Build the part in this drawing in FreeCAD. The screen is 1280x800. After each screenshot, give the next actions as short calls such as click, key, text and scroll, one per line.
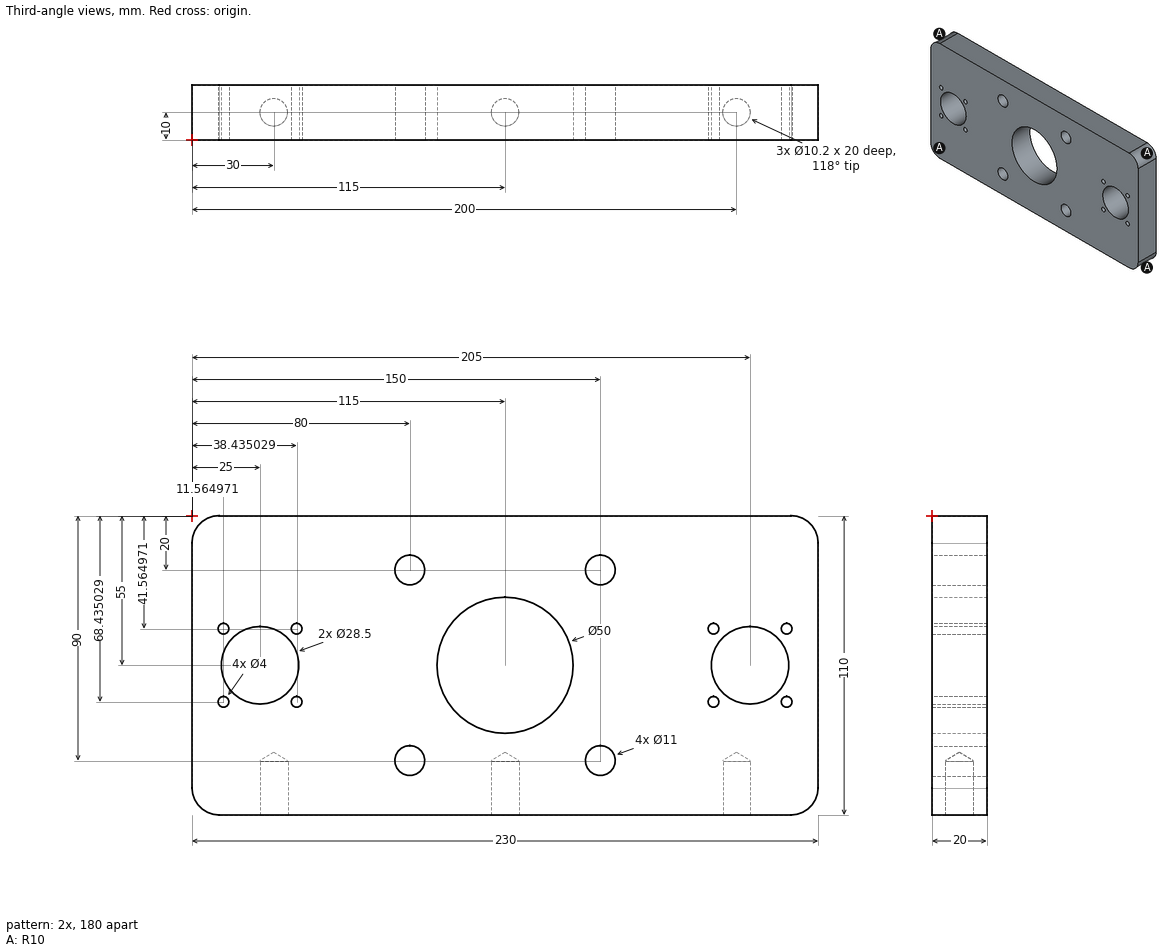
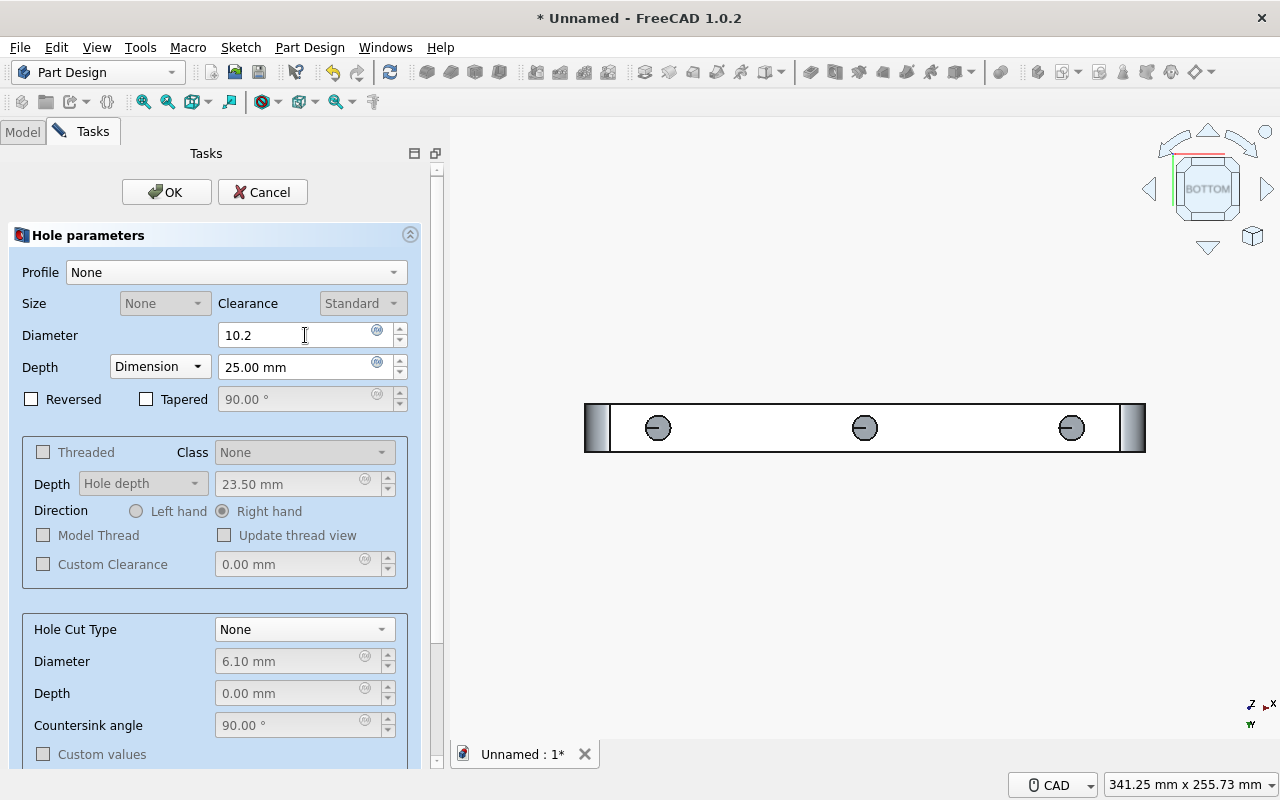
triple_click(305, 367)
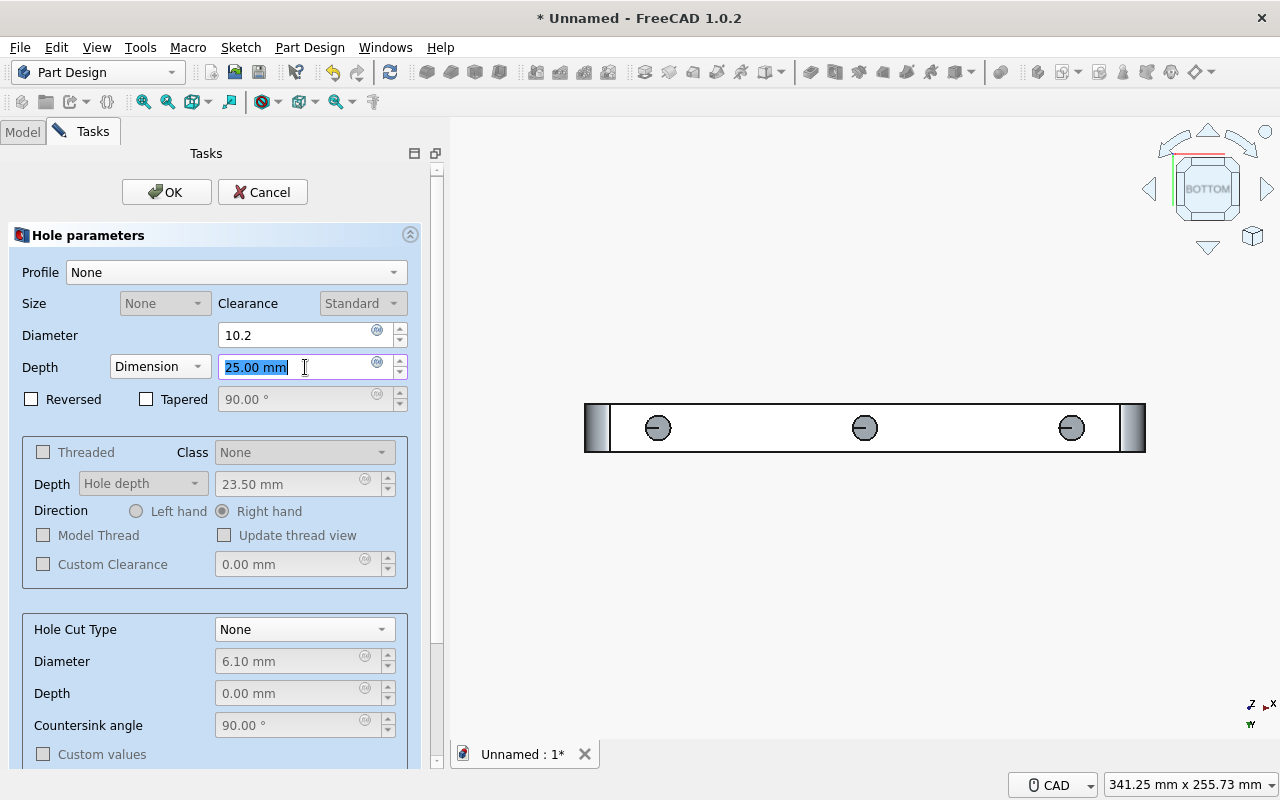
text(20)
key(Tab)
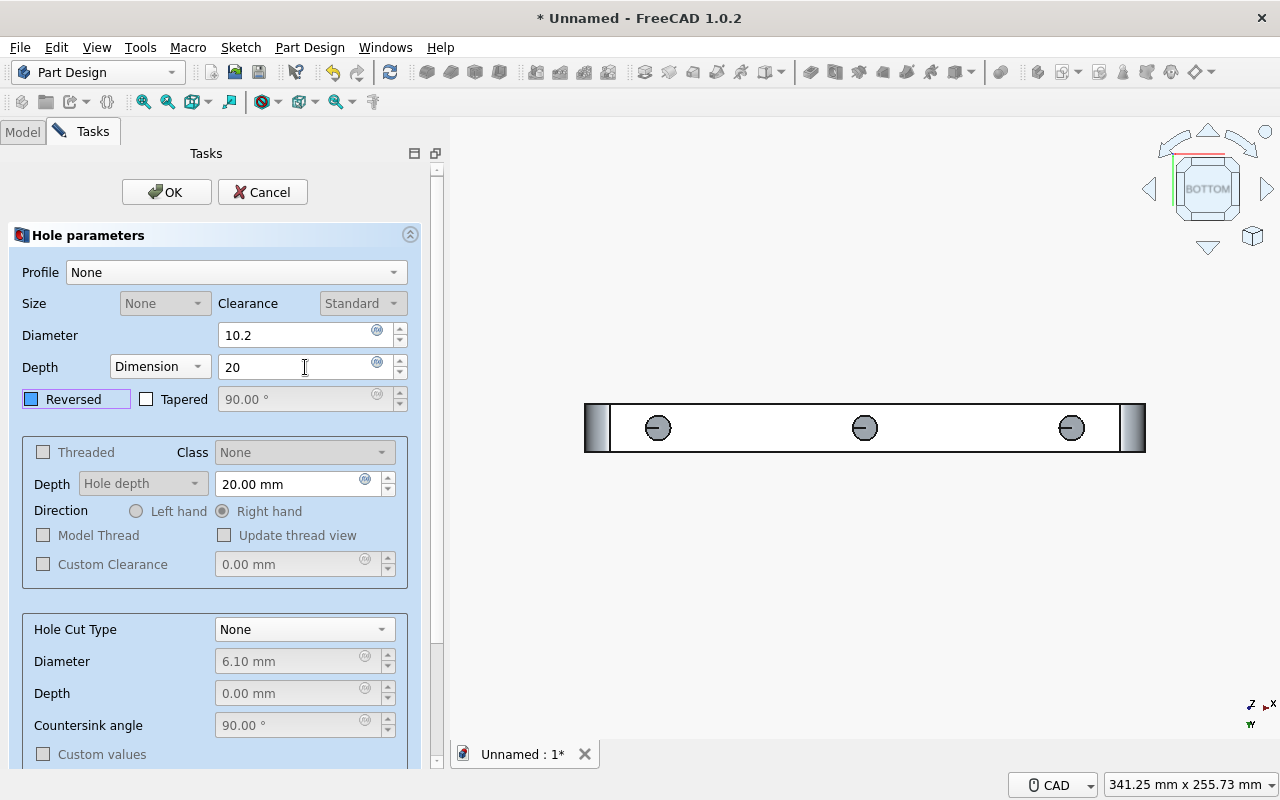
click(167, 192)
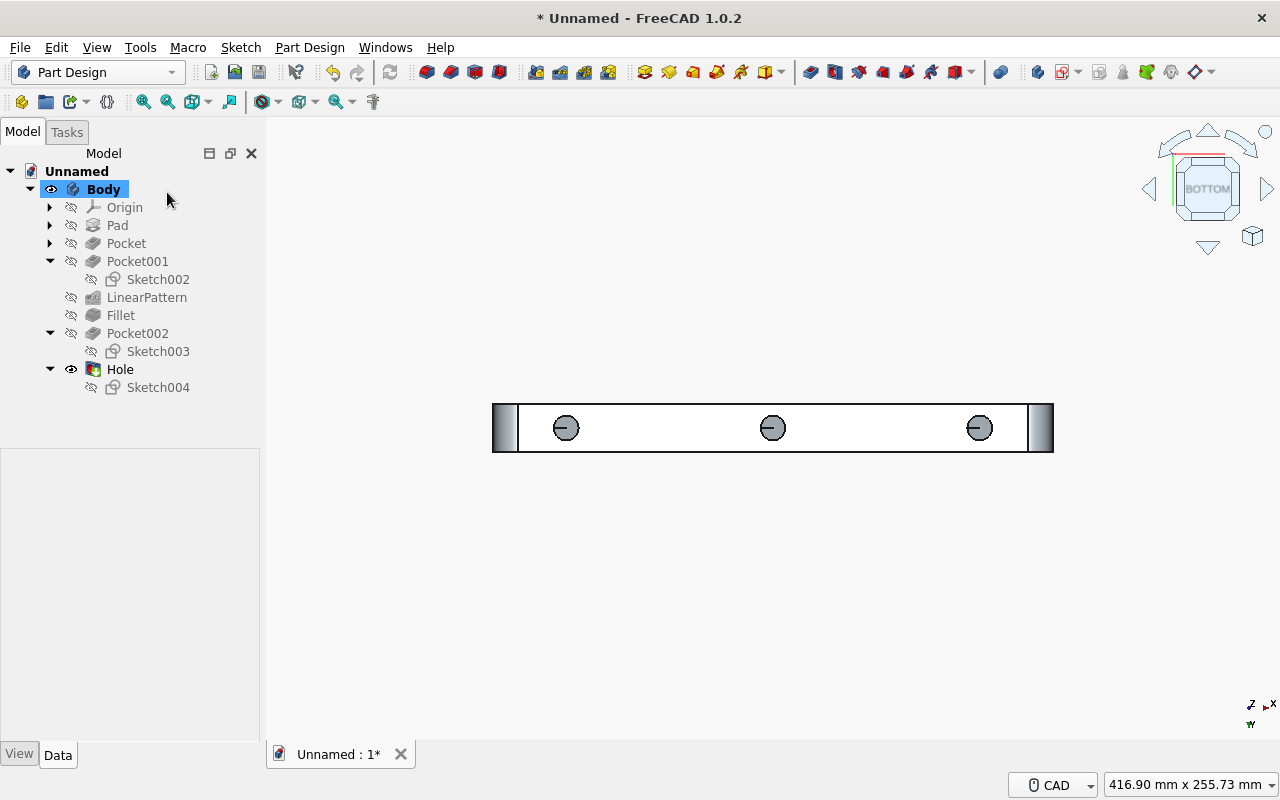
key(0)